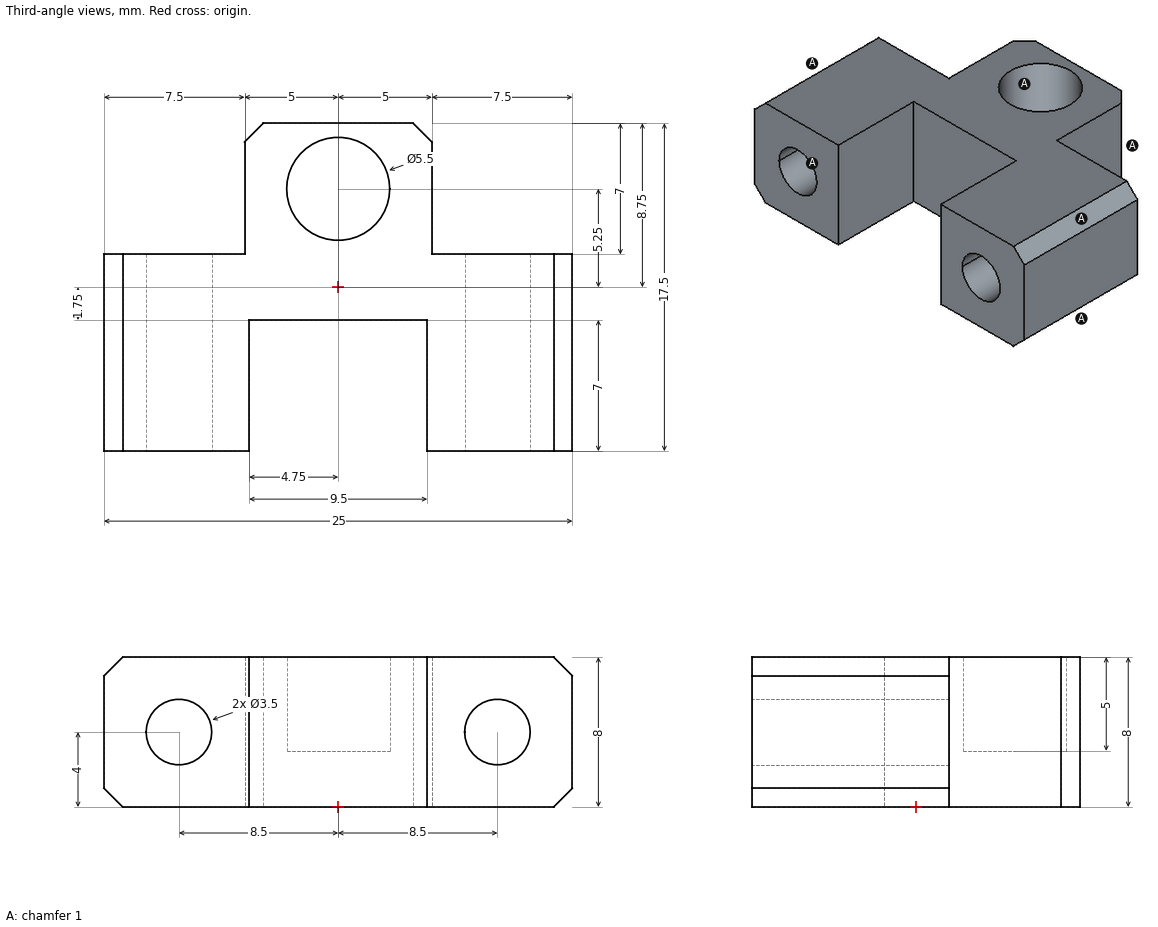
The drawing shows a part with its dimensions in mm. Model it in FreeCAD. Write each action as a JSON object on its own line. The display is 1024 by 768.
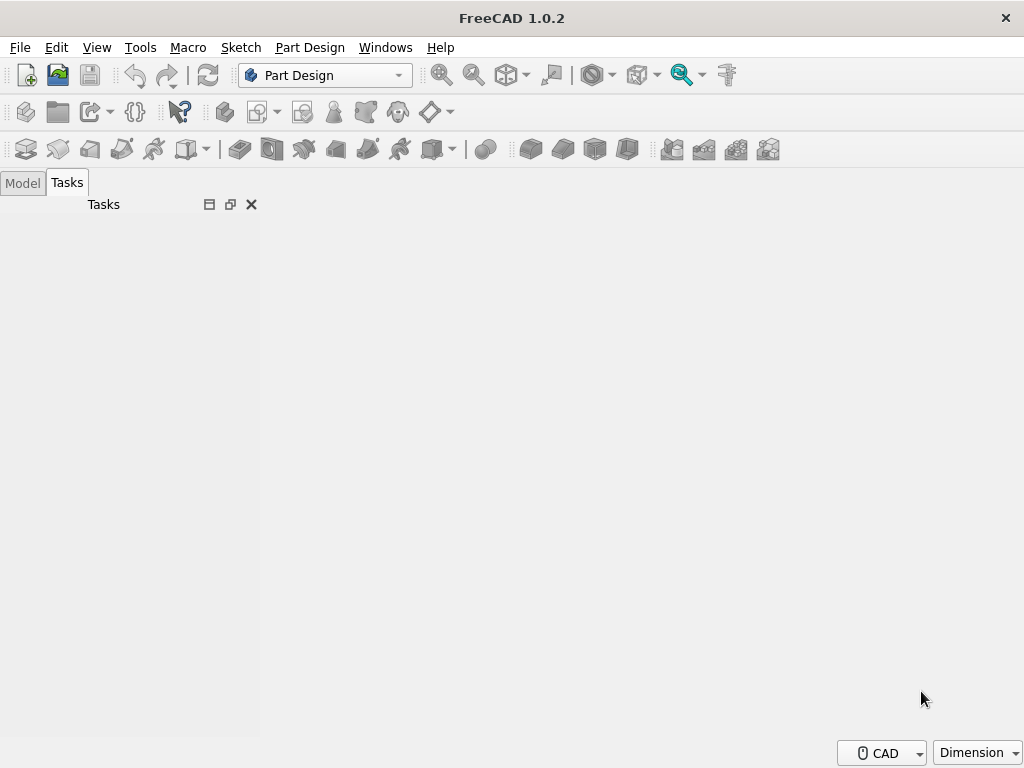
{"action": "left_click", "coordinate": [26, 76]}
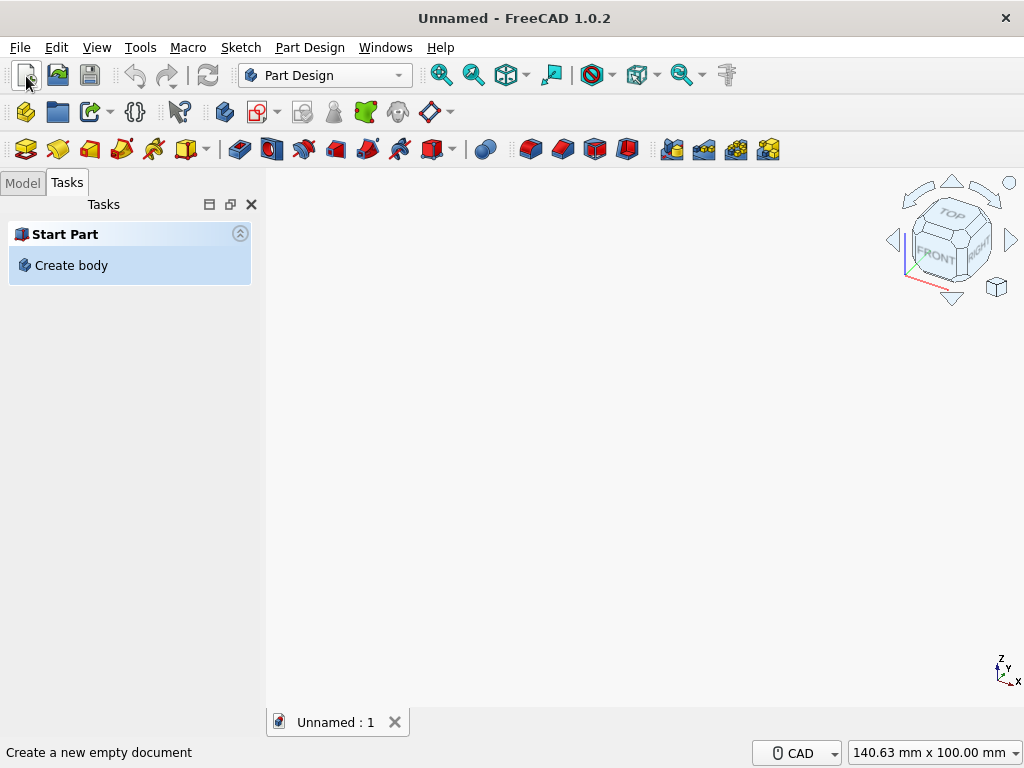
{"action": "left_click", "coordinate": [258, 112]}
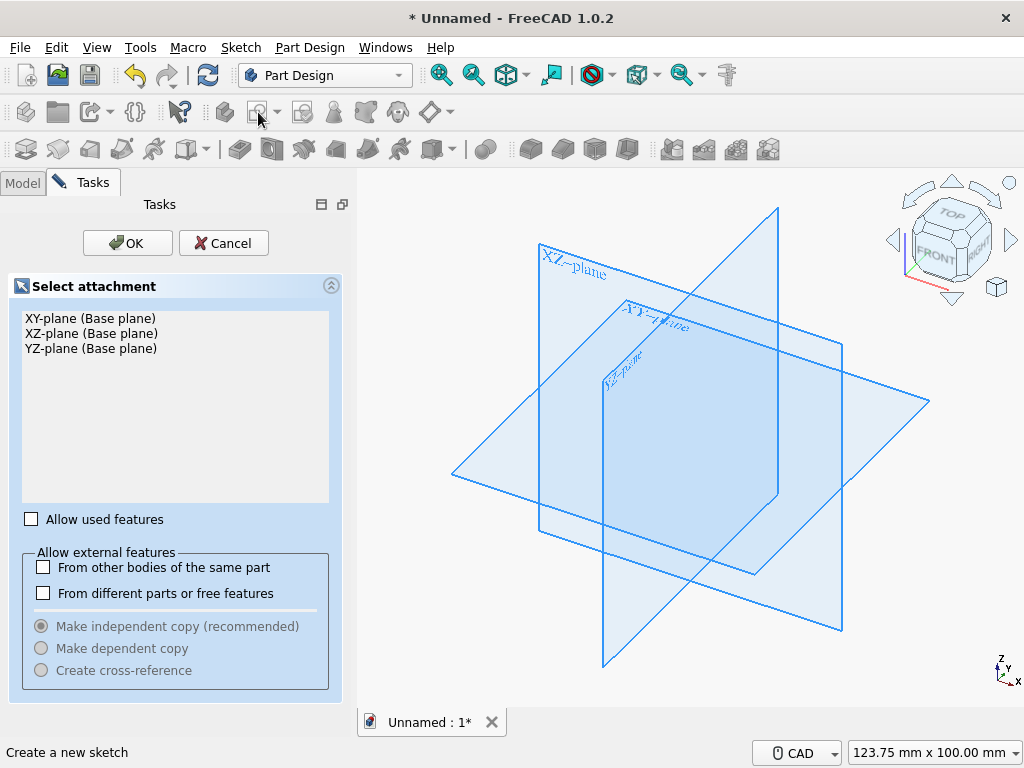
{"action": "left_click", "coordinate": [82, 318]}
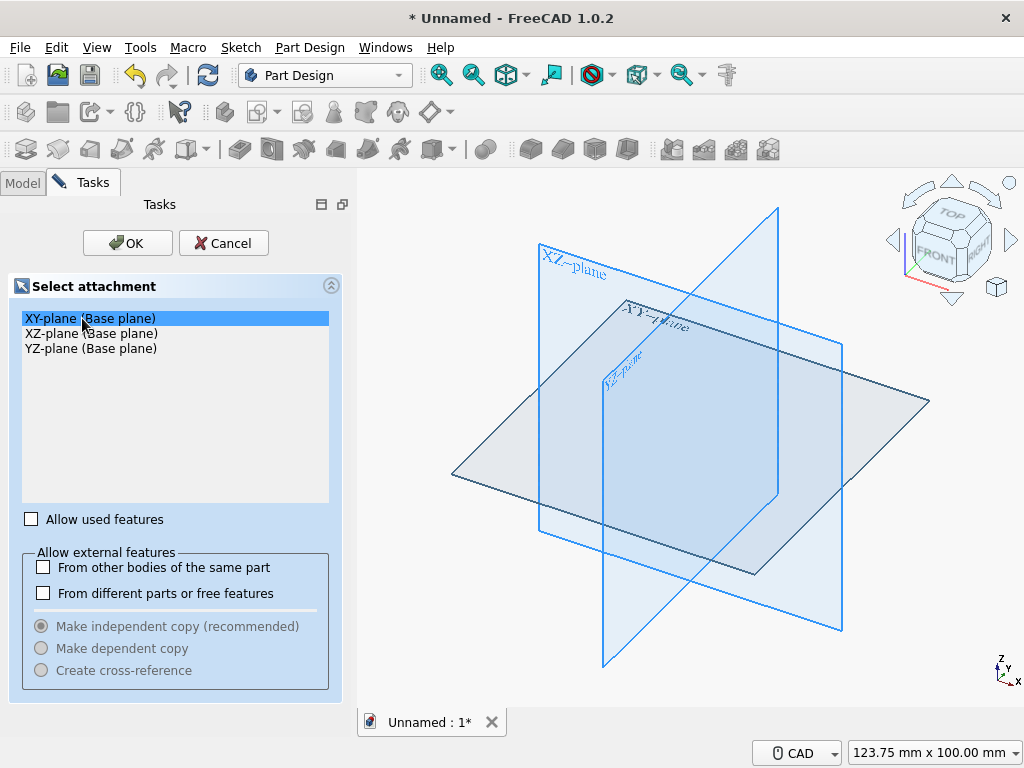
{"action": "left_click", "coordinate": [128, 243]}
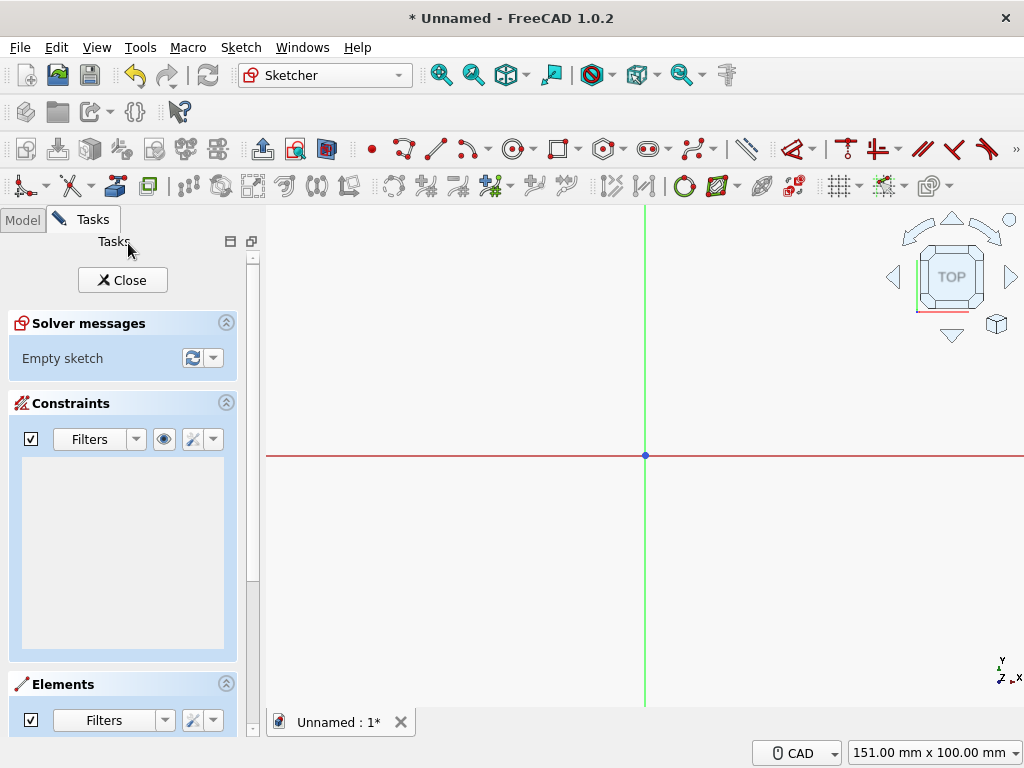
{"action": "scroll", "coordinate": [675, 456], "scroll_direction": "up", "scroll_amount": 6}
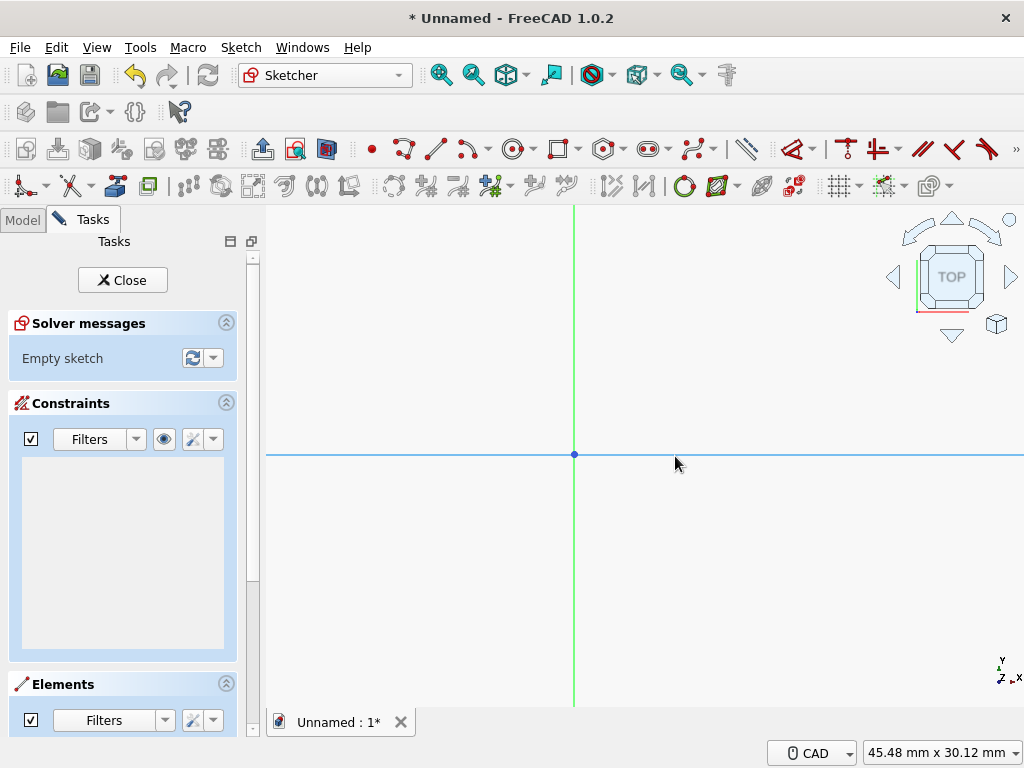
{"action": "key", "text": "g v"}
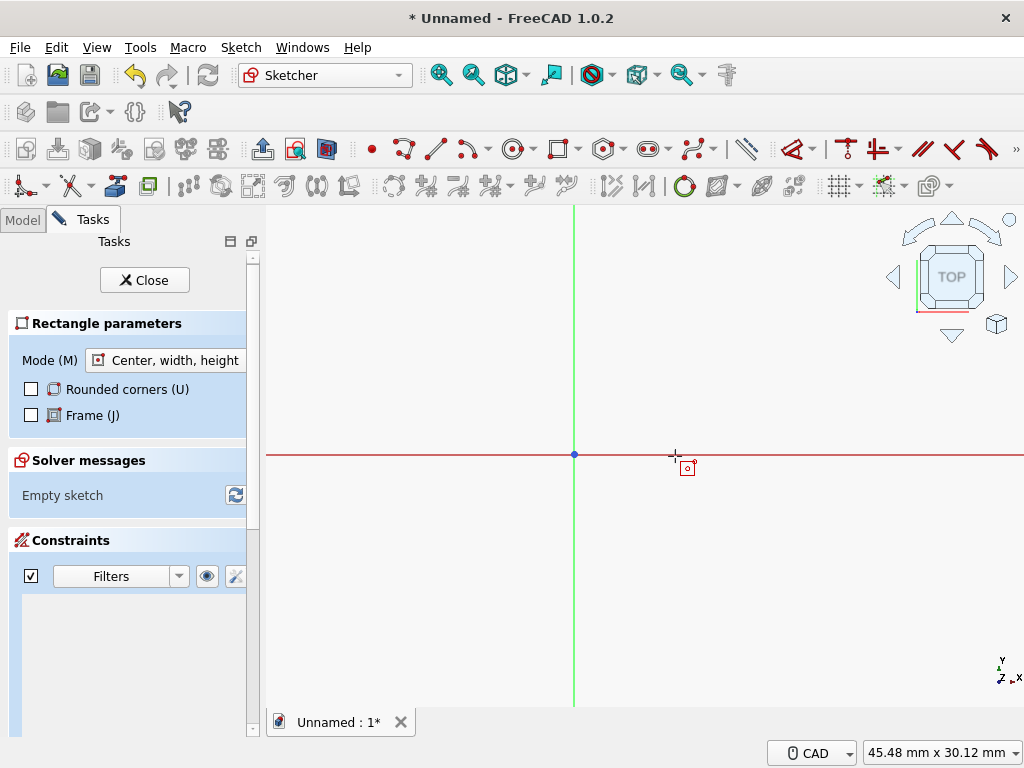
{"action": "left_click", "coordinate": [574, 455]}
{"action": "mouse_move", "coordinate": [782, 309]}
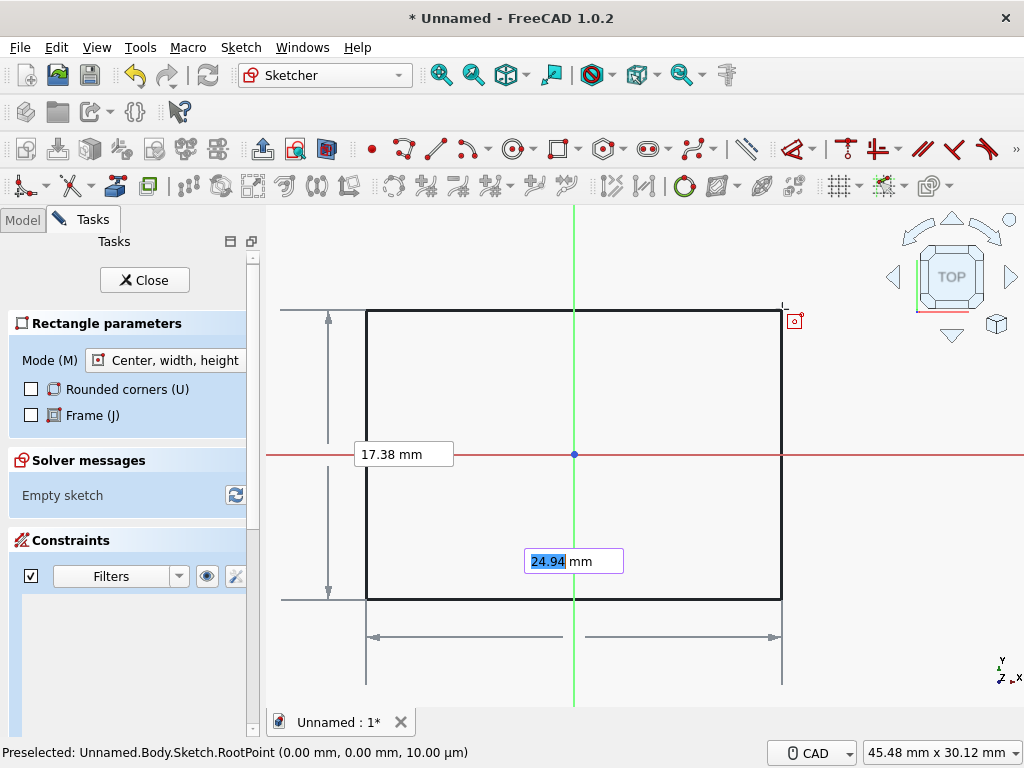
{"action": "type", "text": "25"}
{"action": "key", "text": "Tab"}
{"action": "type", "text": "17.5"}
{"action": "key", "text": "Return"}
{"action": "key", "text": "Escape"}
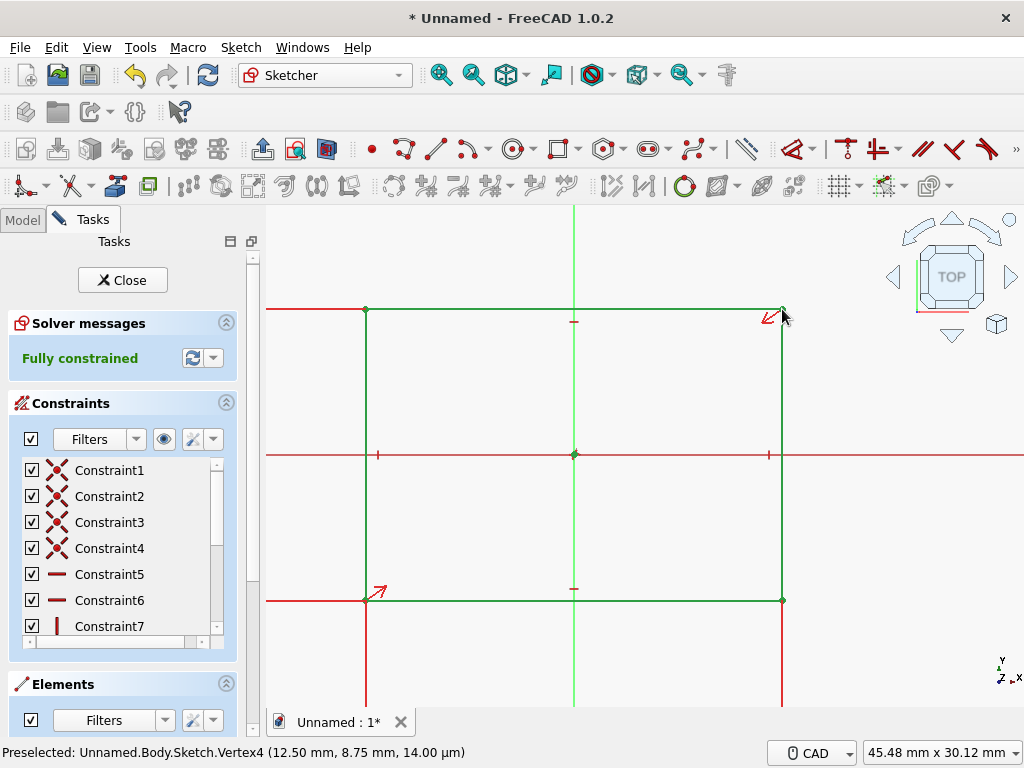
{"action": "left_click", "coordinate": [123, 280]}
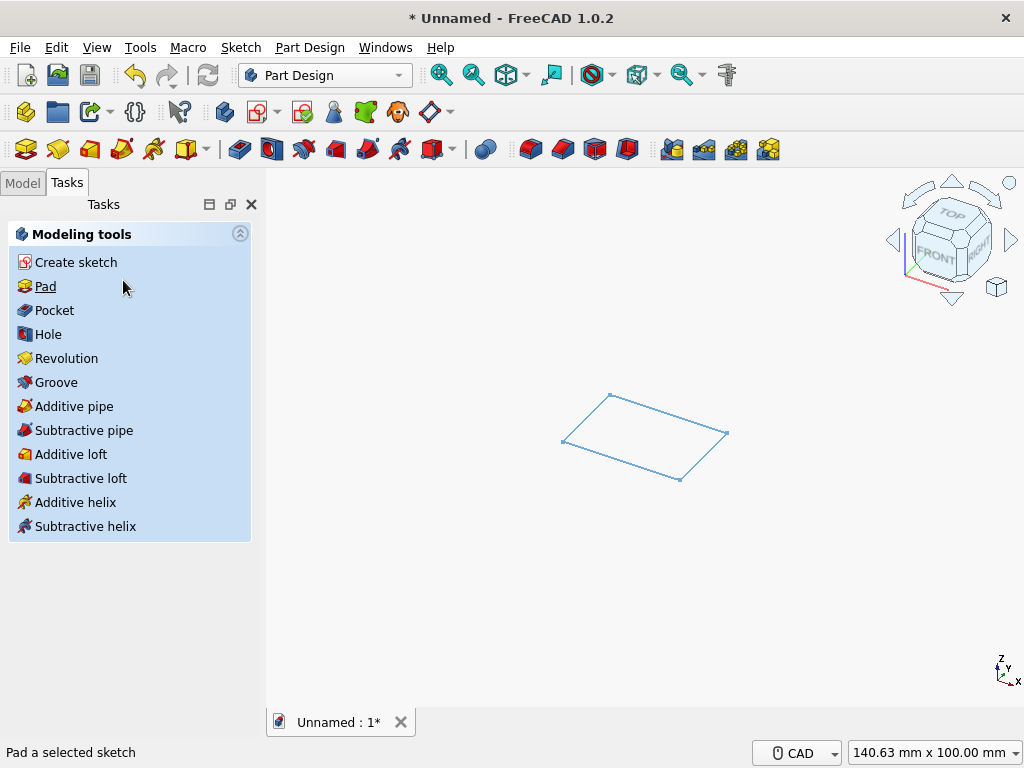
{"action": "left_click", "coordinate": [26, 150]}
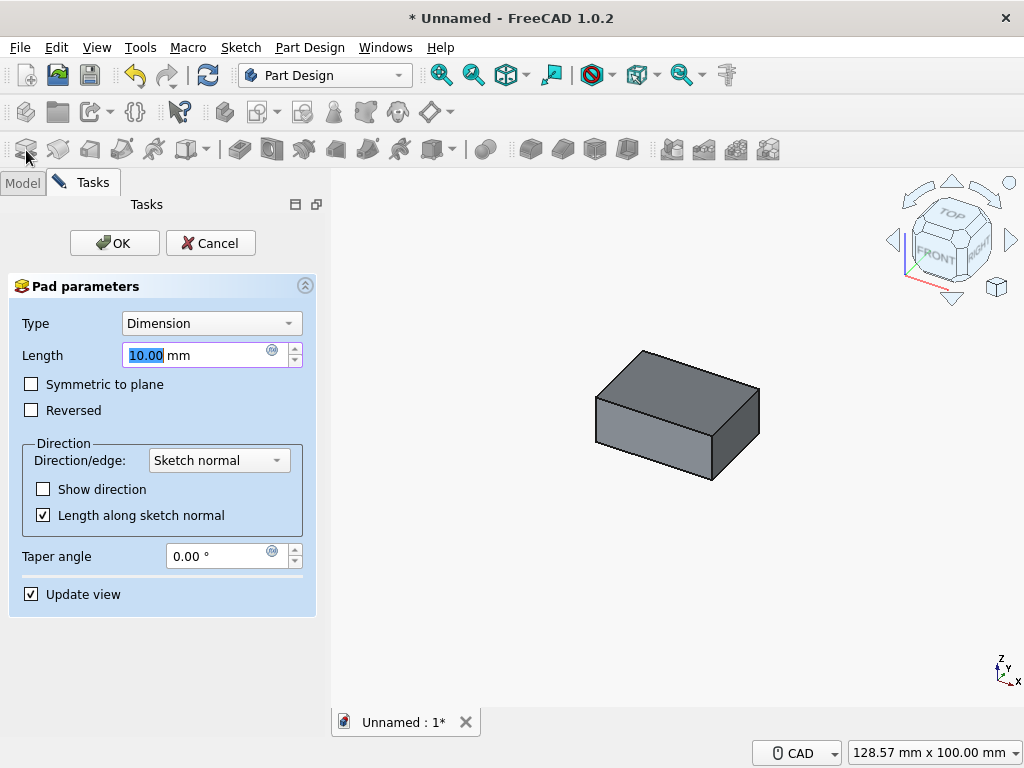
{"action": "type", "text": "8"}
{"action": "key", "text": "Tab"}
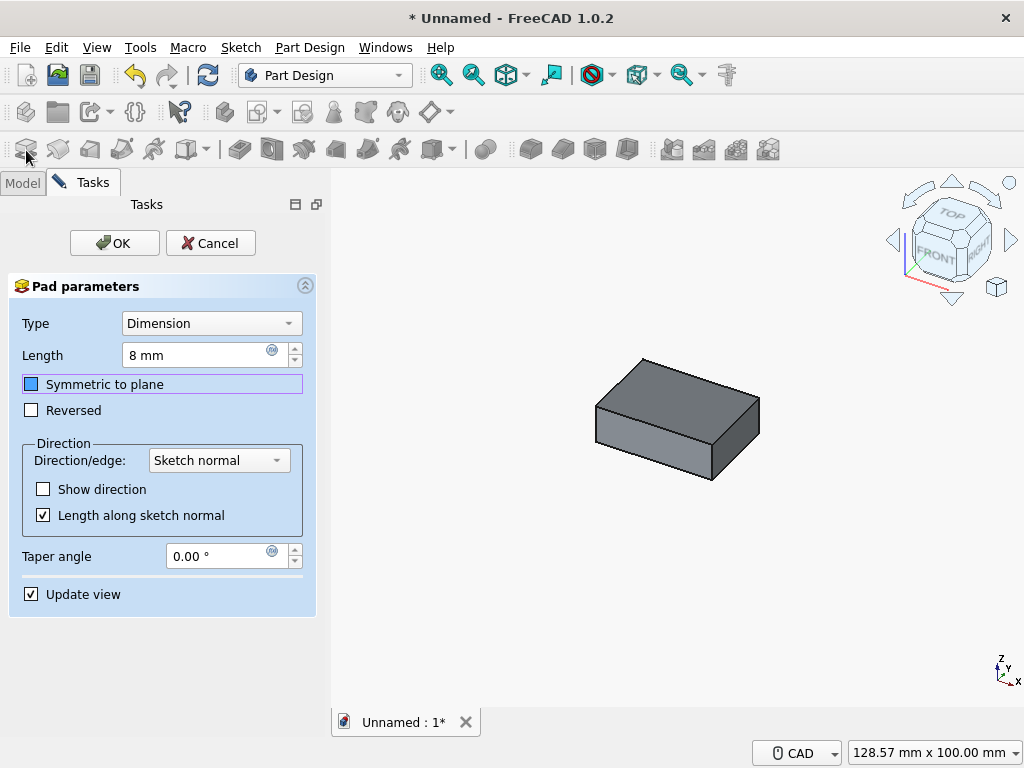
{"action": "left_click", "coordinate": [115, 243]}